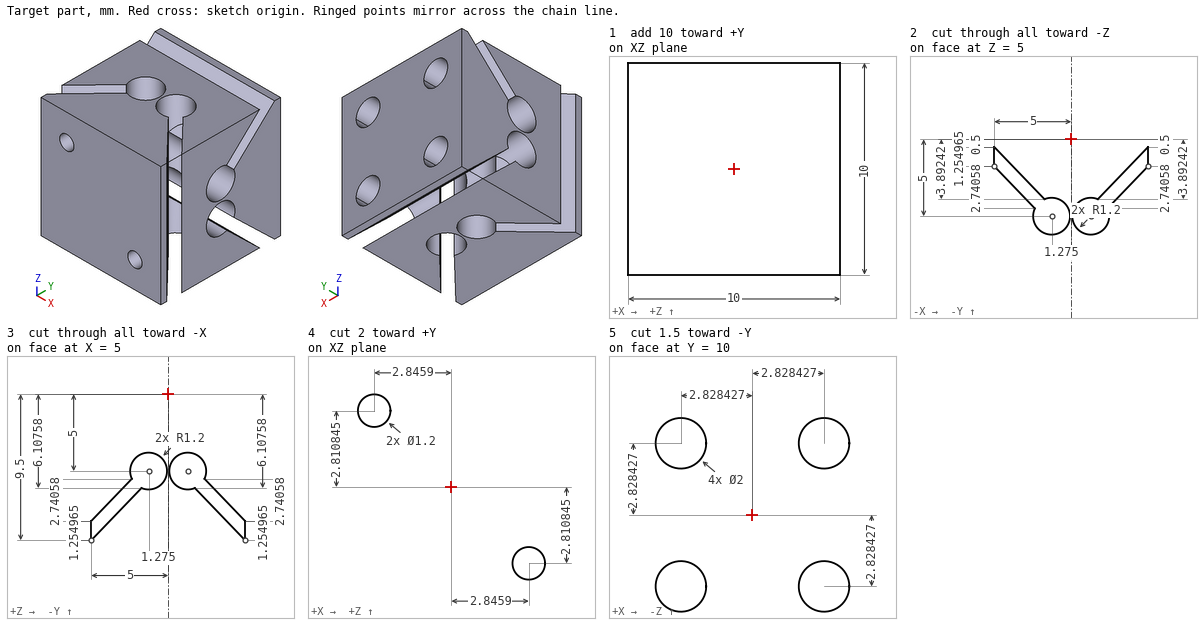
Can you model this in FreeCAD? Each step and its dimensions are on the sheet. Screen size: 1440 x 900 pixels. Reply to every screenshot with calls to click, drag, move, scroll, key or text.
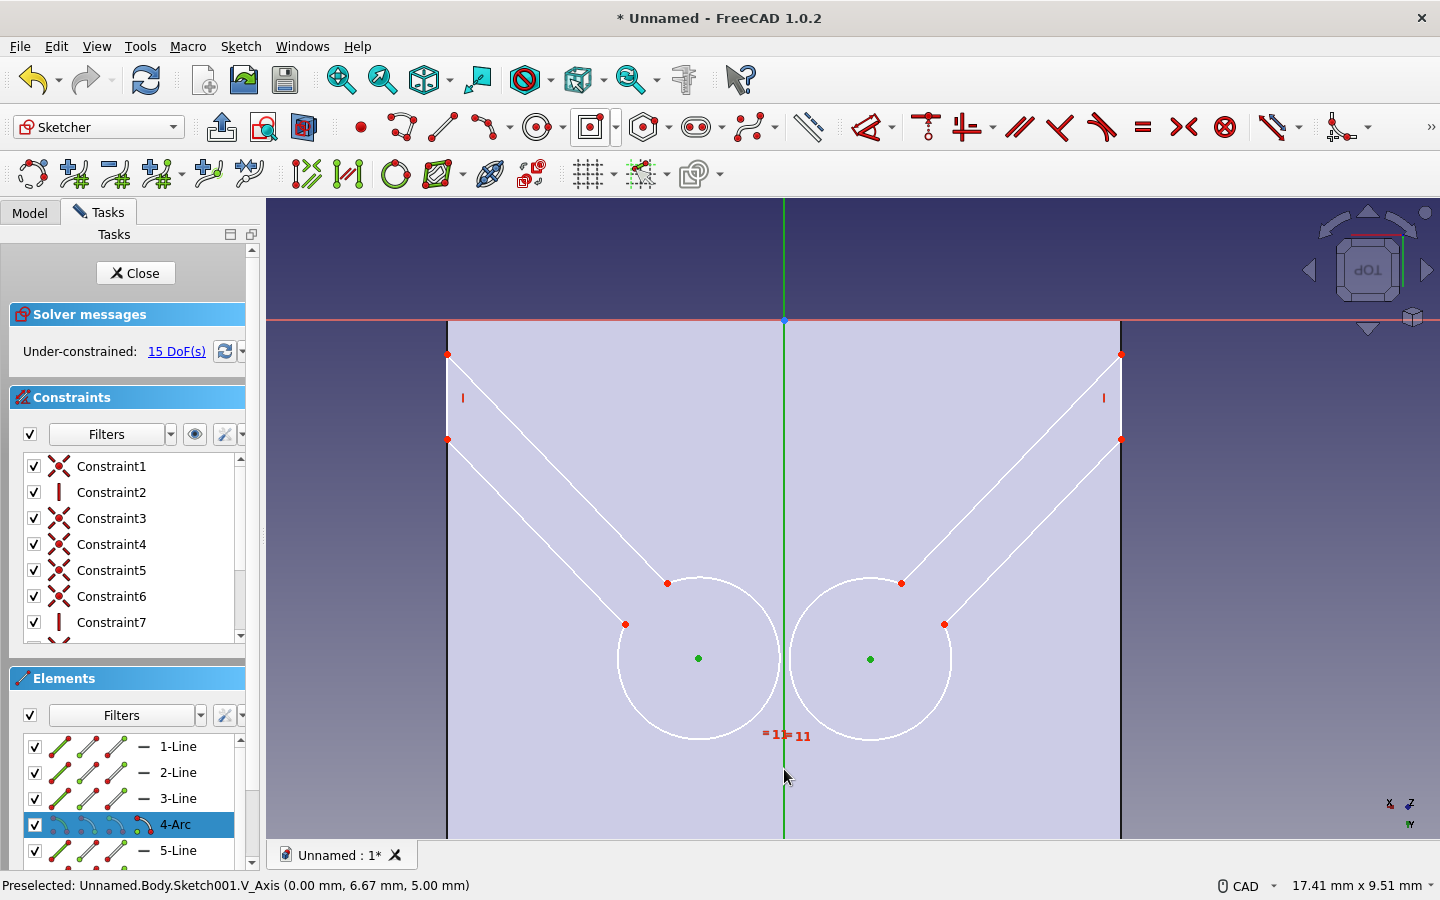
click(1184, 128)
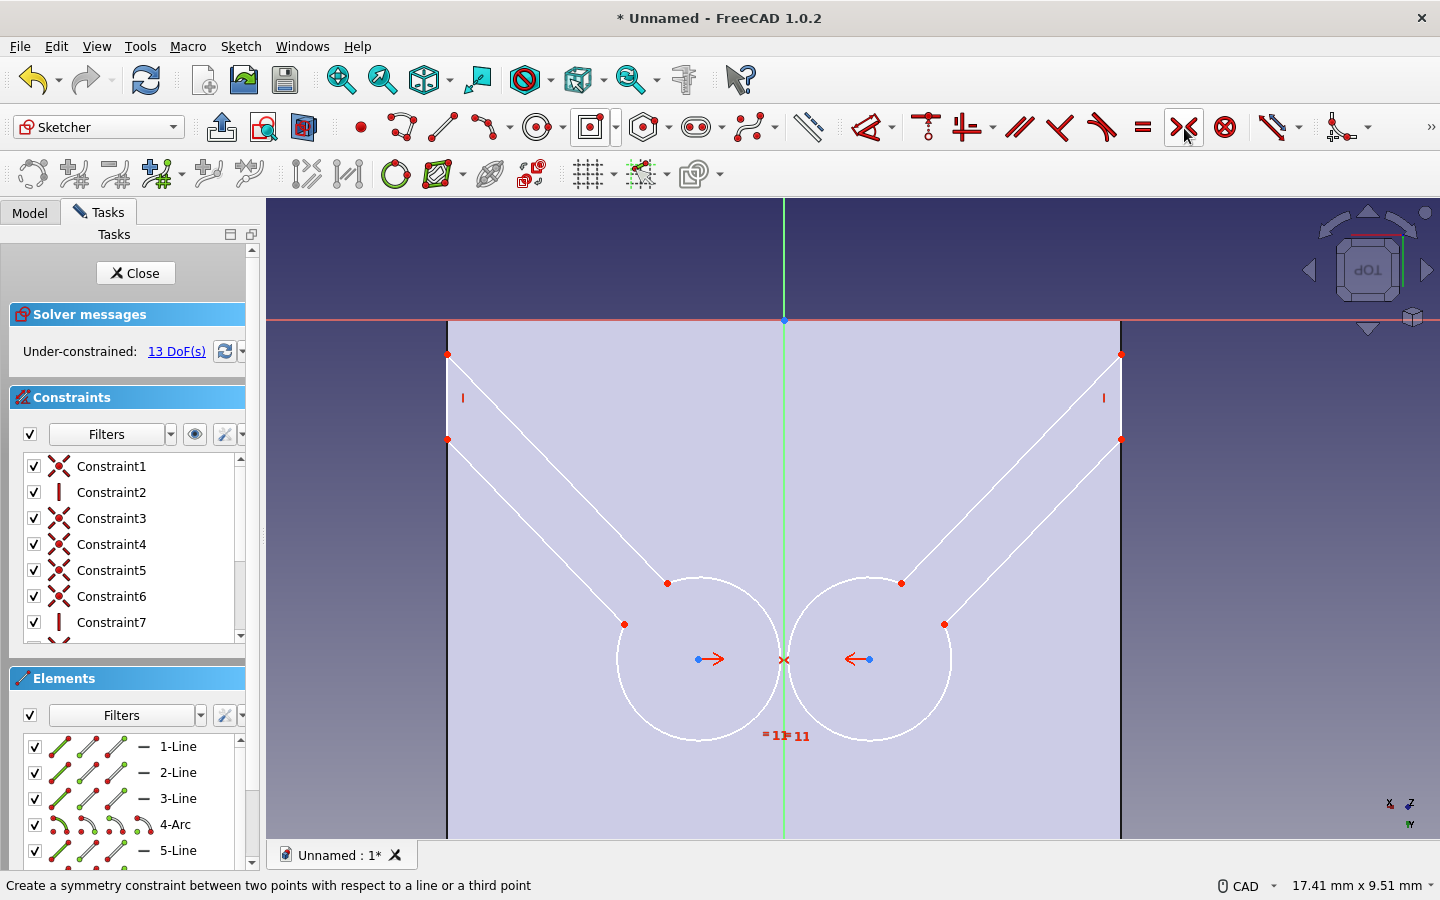
click(447, 440)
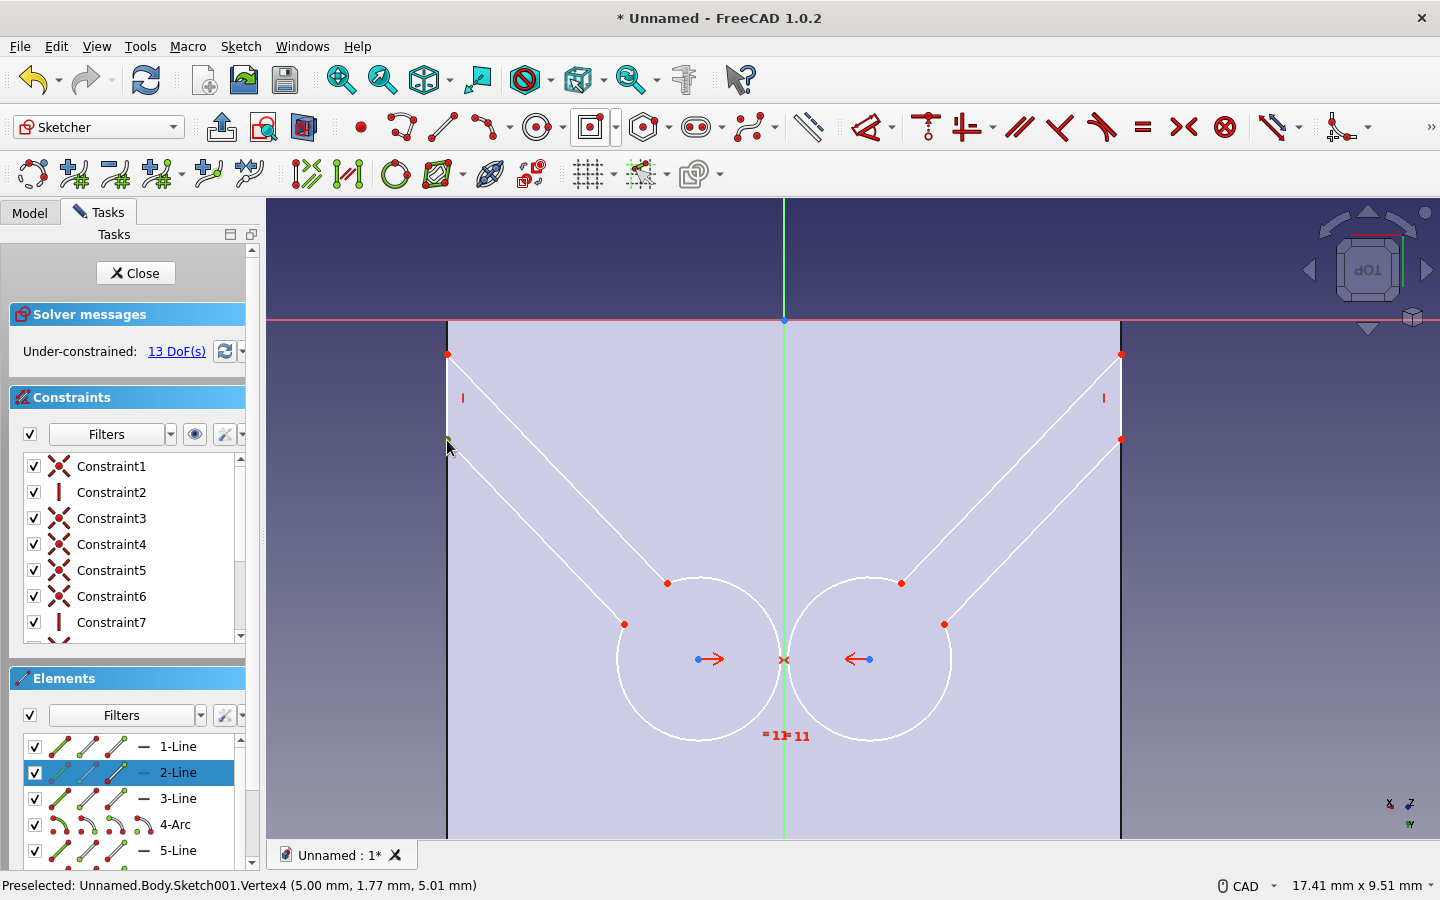
click(1121, 440)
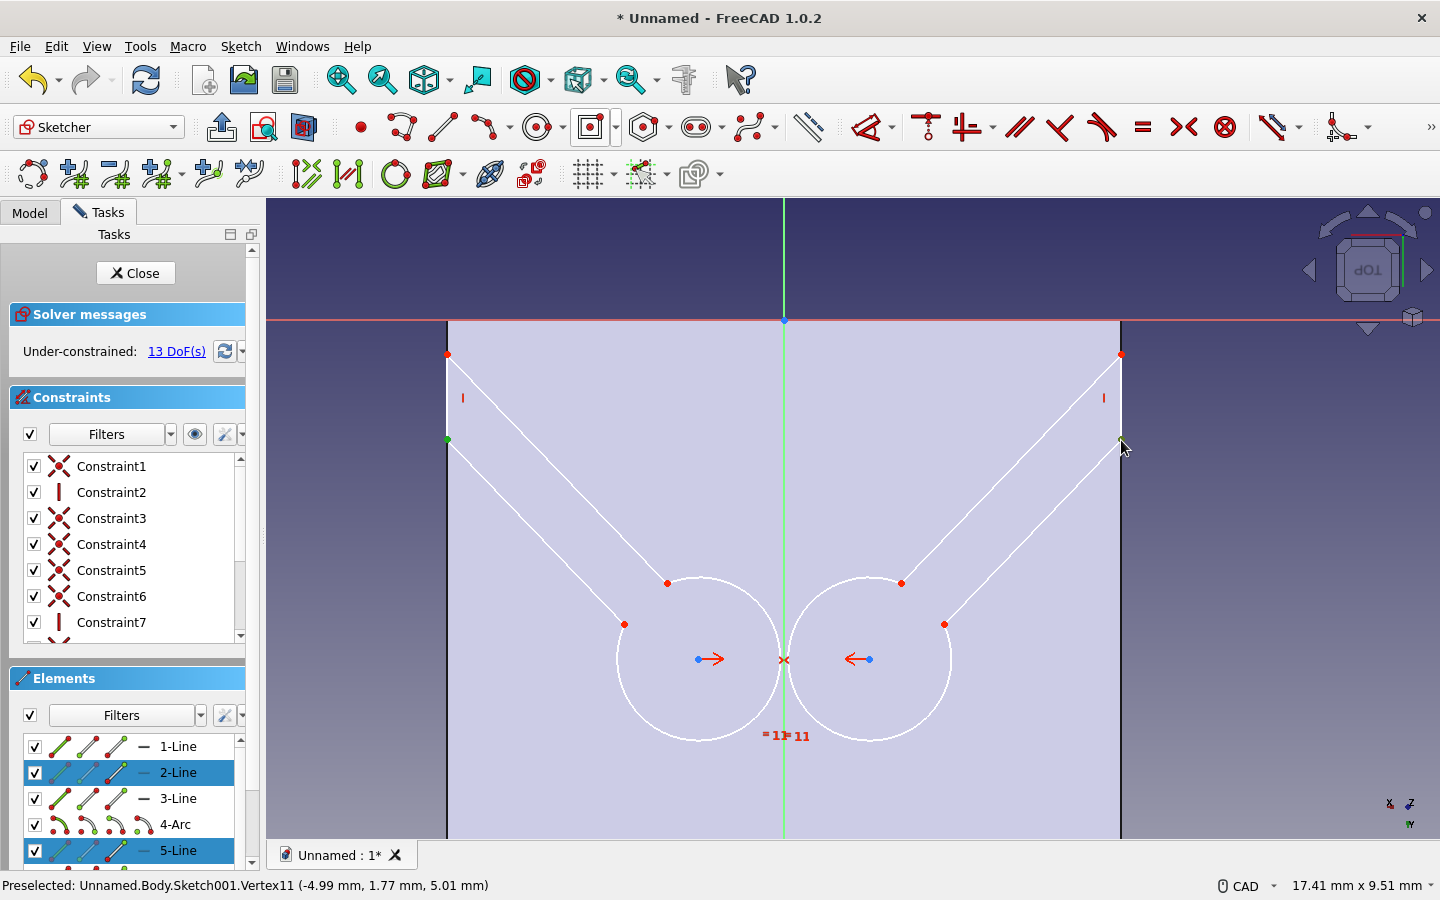
click(784, 769)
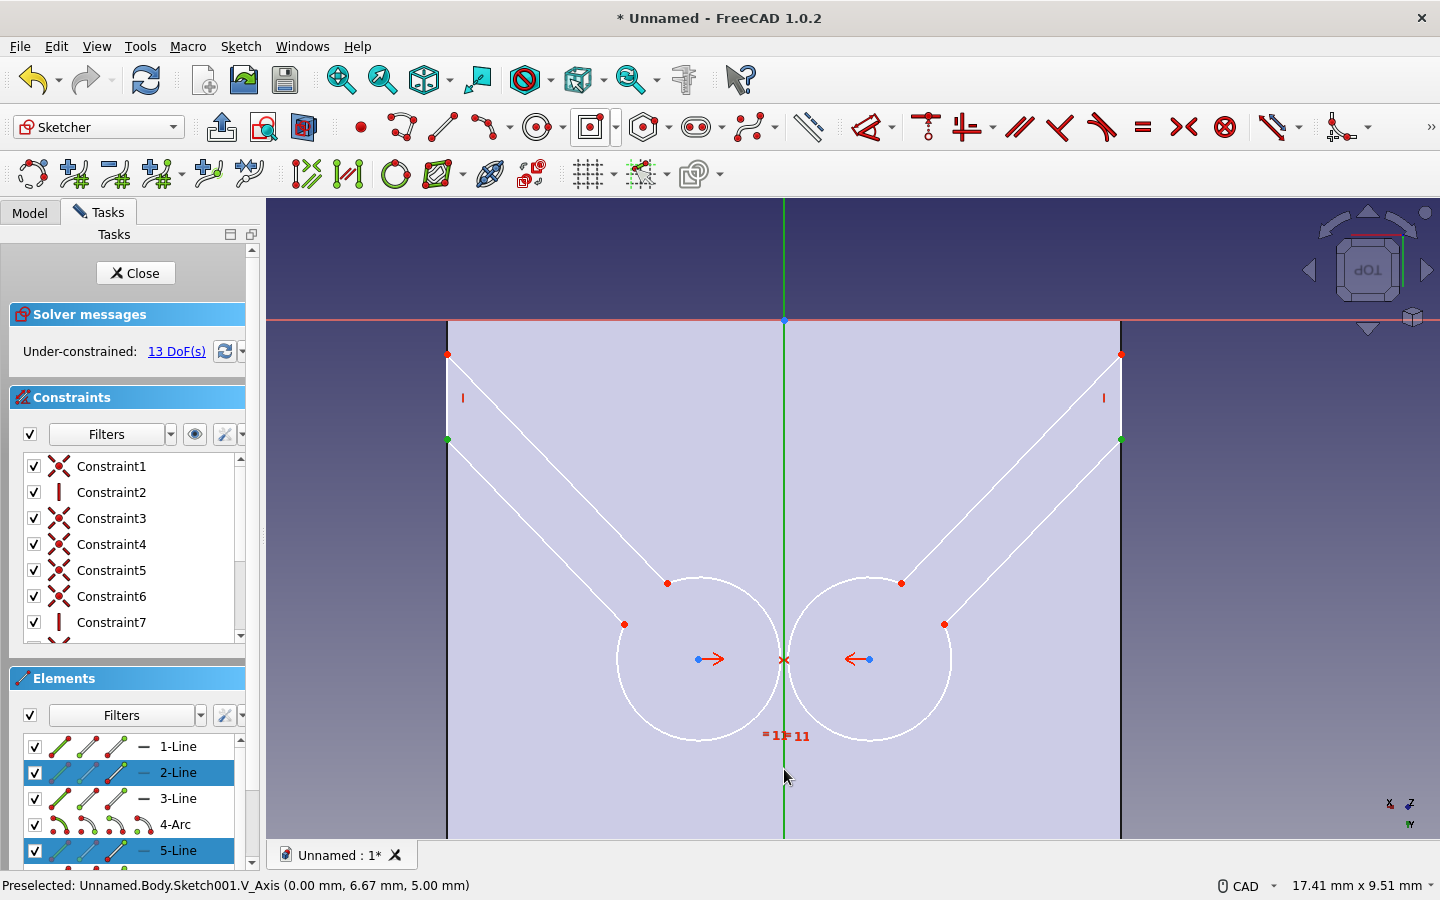
click(1184, 128)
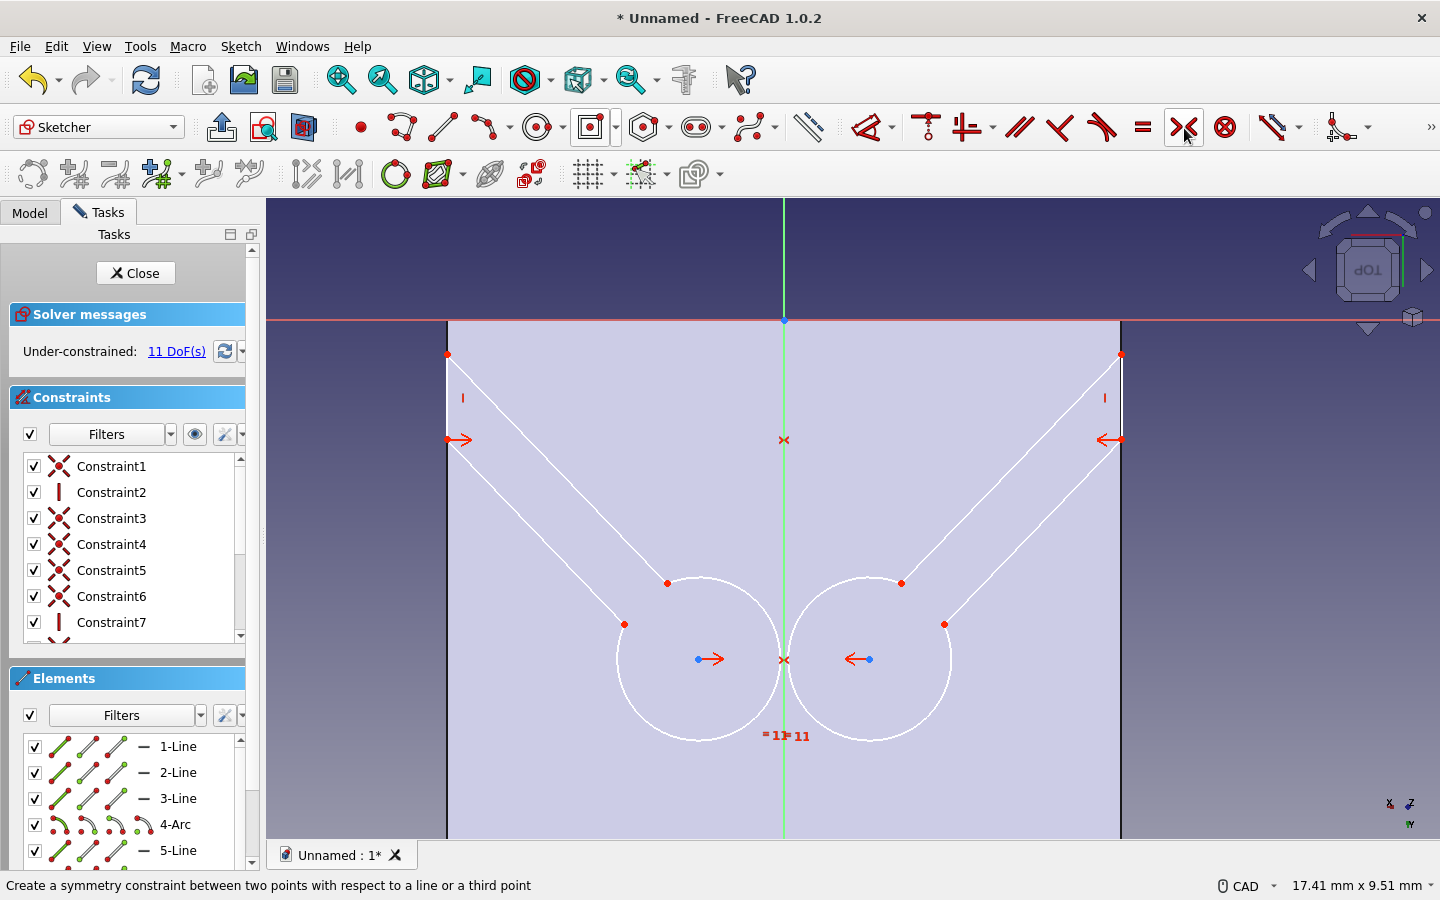
click(866, 128)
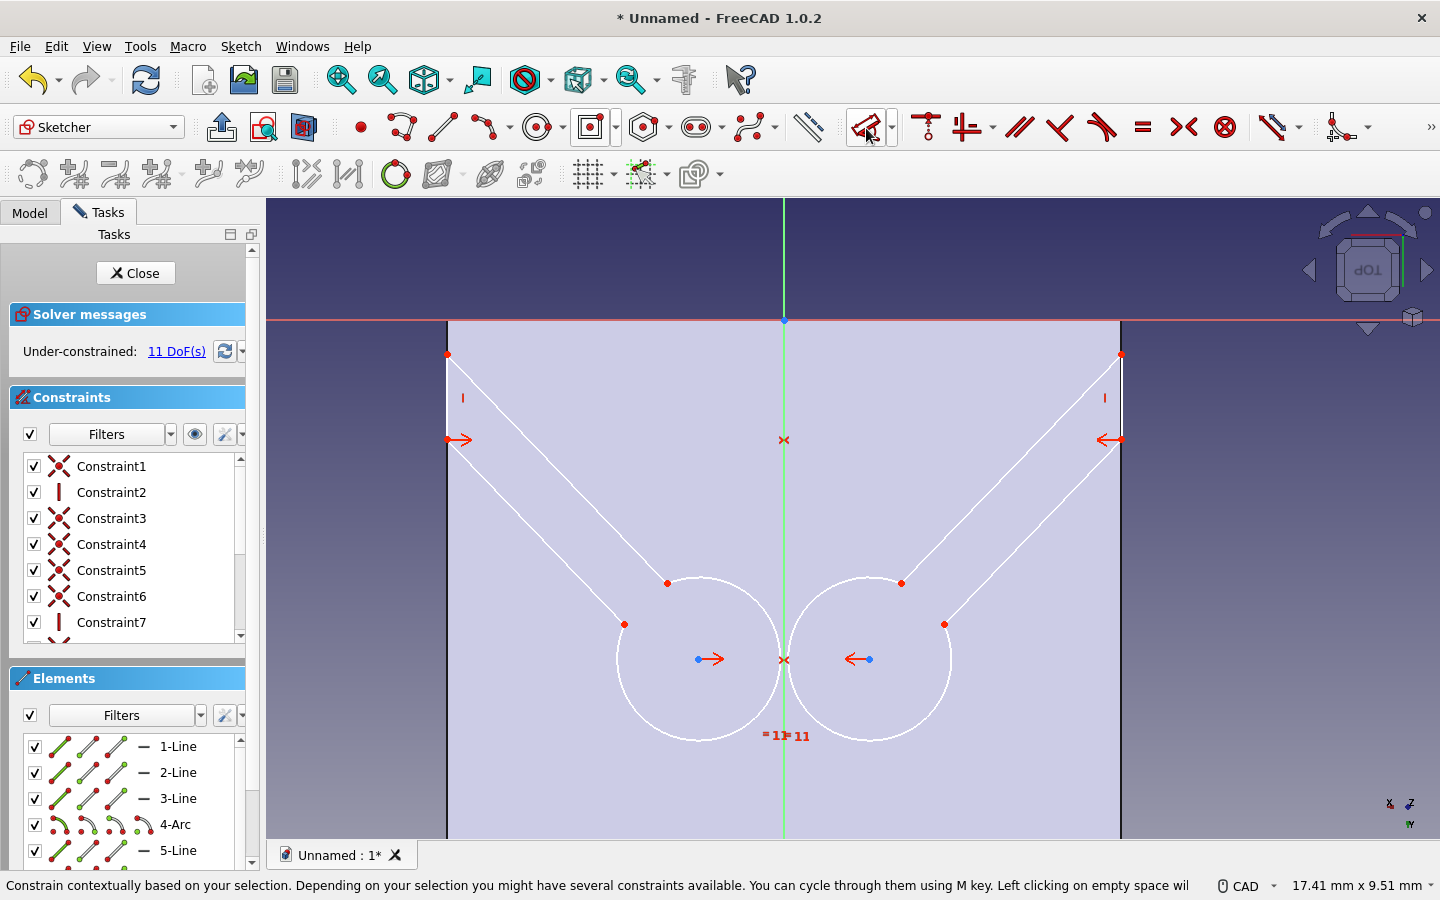
click(672, 736)
click(661, 766)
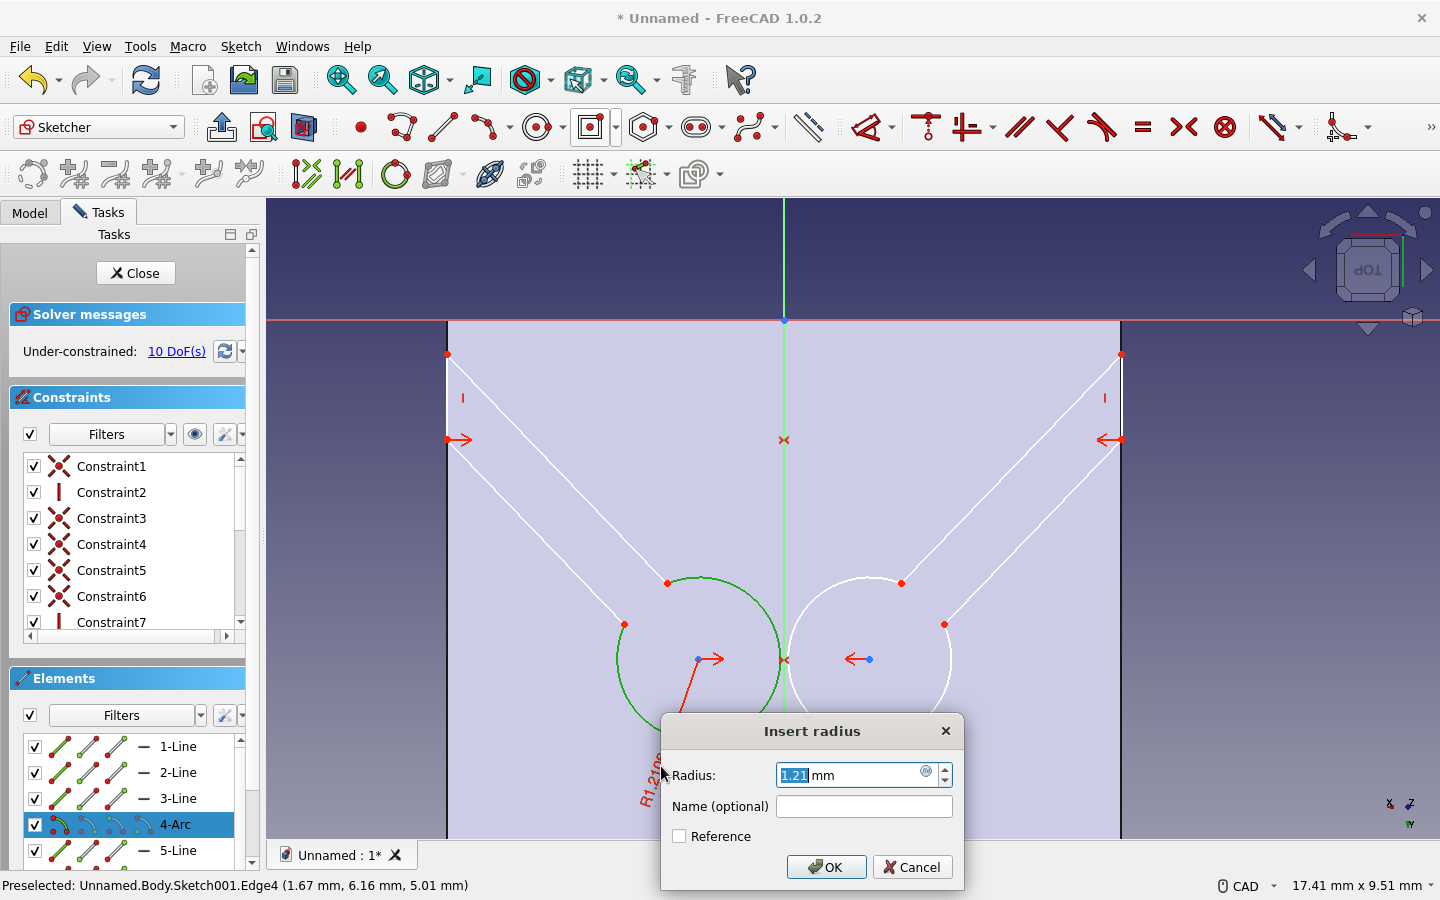
text(1.2)
key(Return)